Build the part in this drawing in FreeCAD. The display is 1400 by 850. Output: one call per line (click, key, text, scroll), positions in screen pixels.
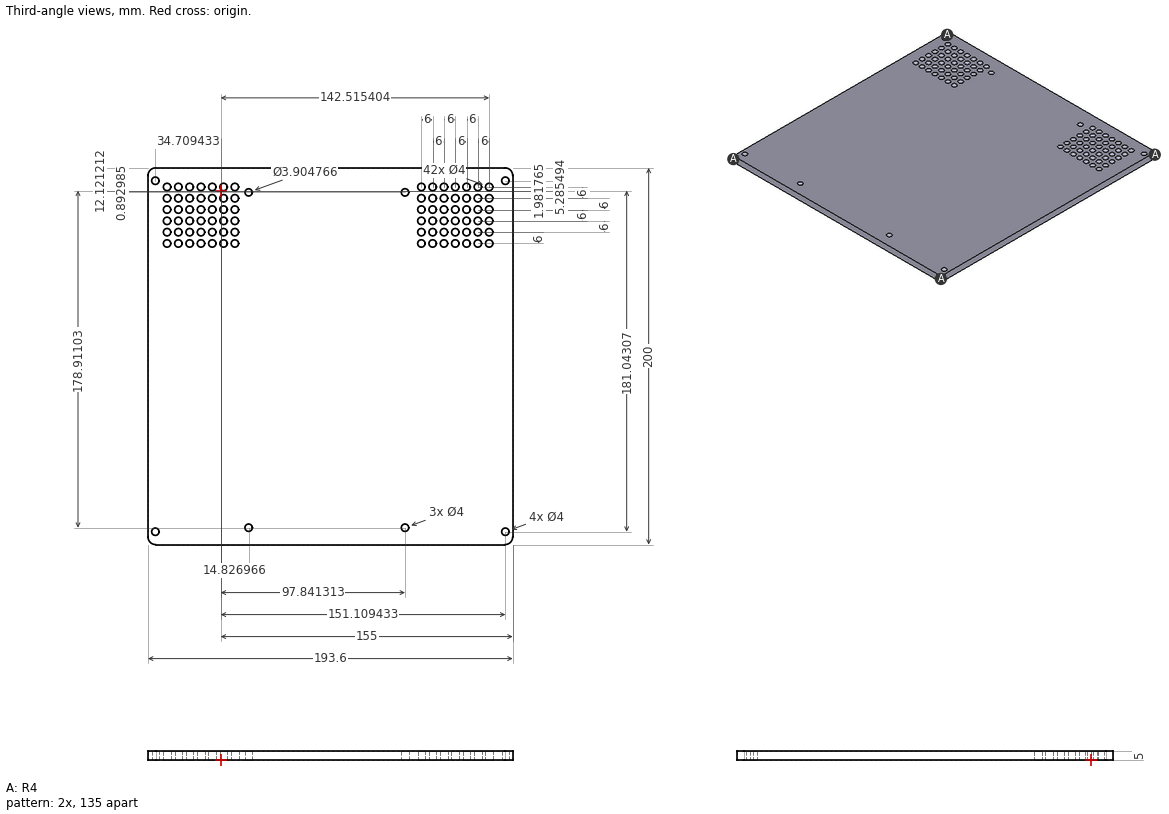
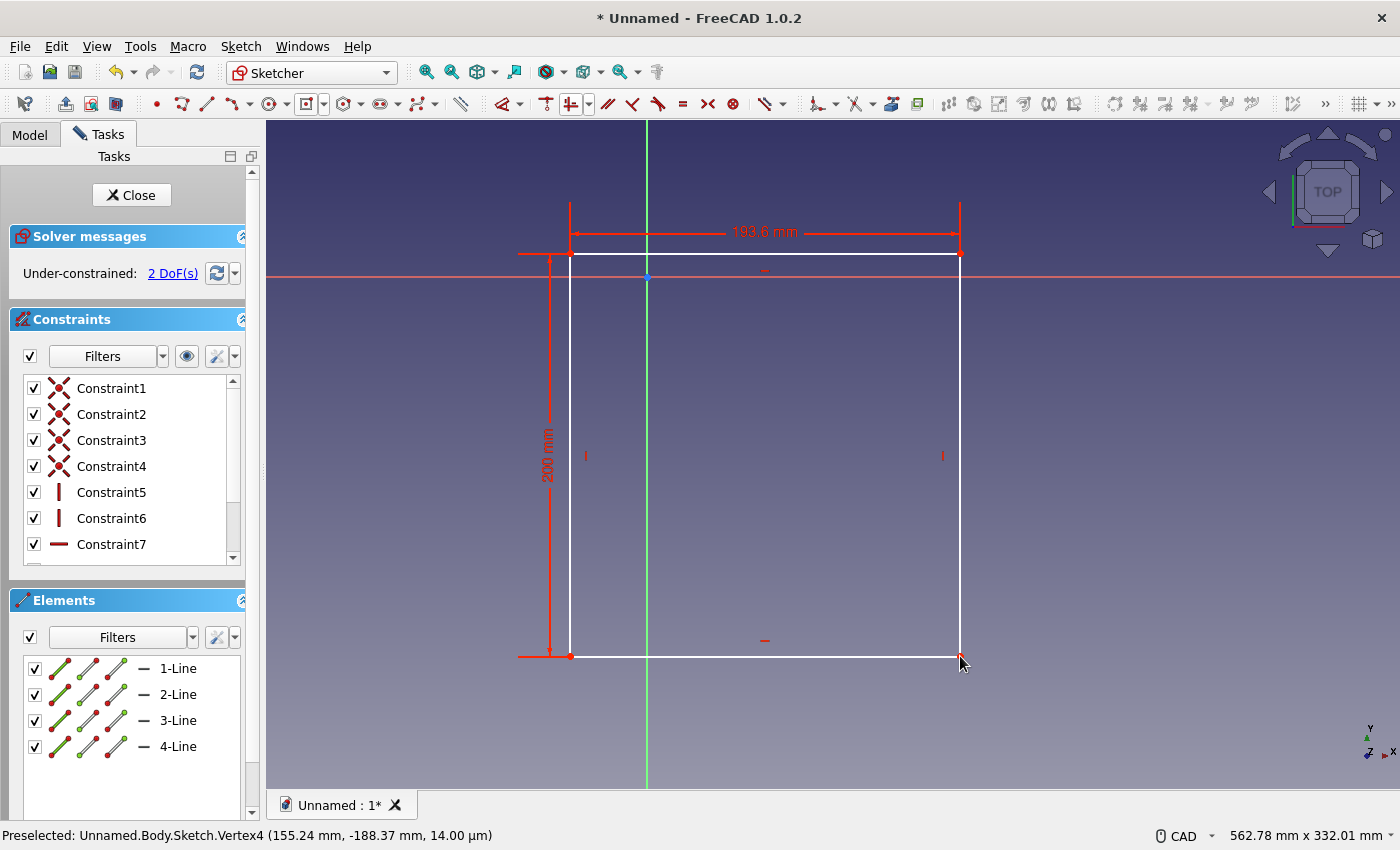
click(502, 104)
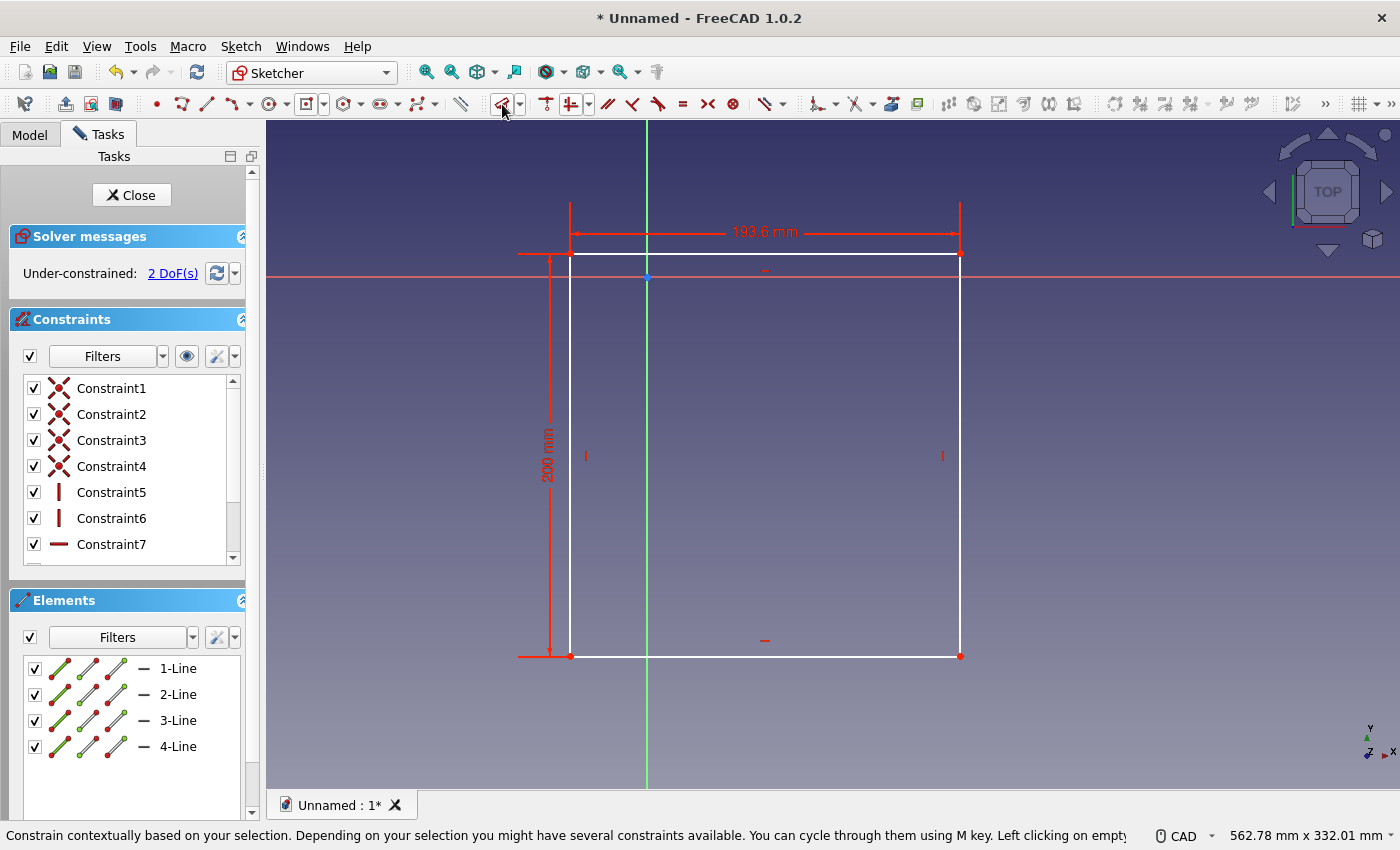
click(960, 657)
click(804, 691)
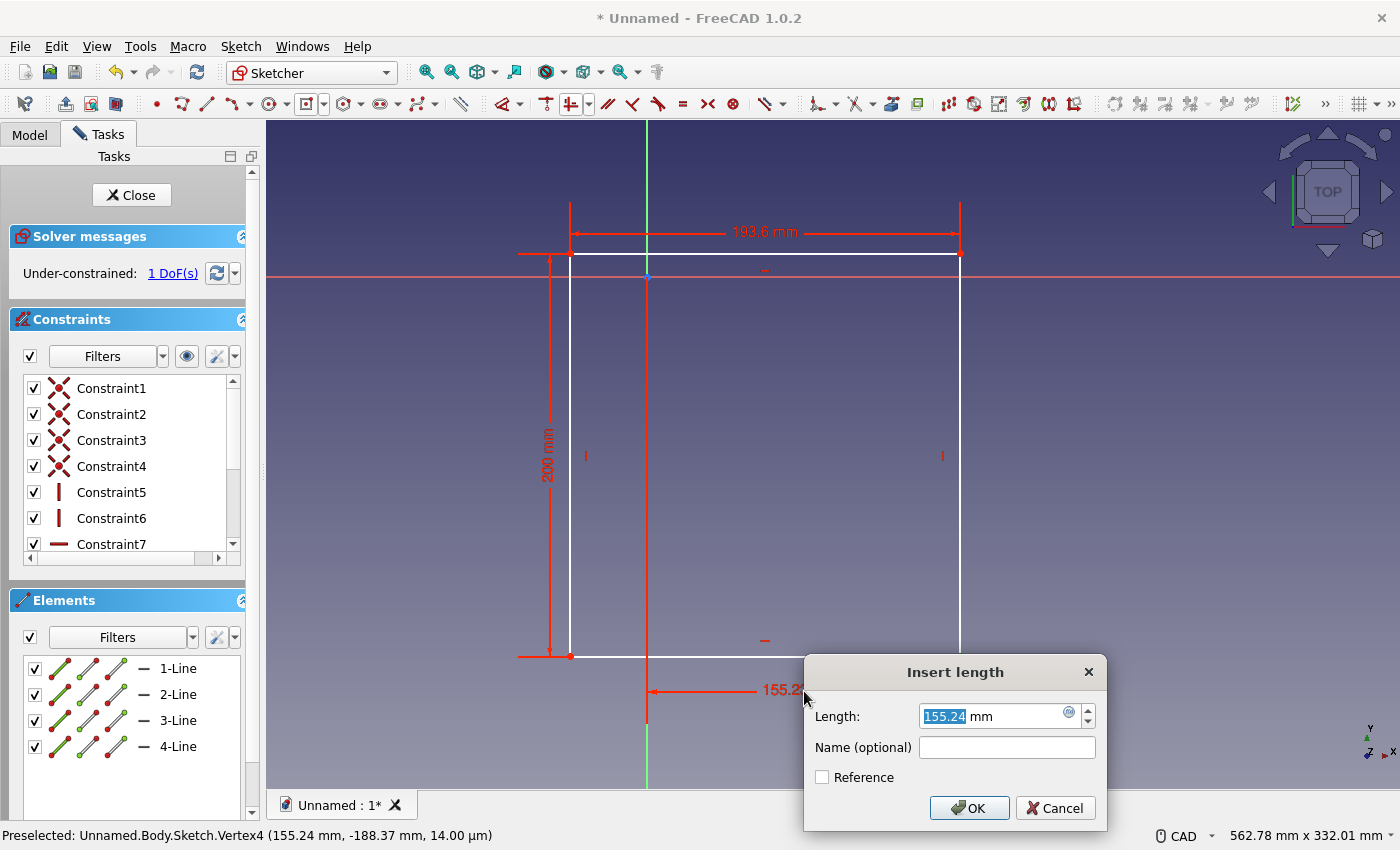
text(155)
key(Return)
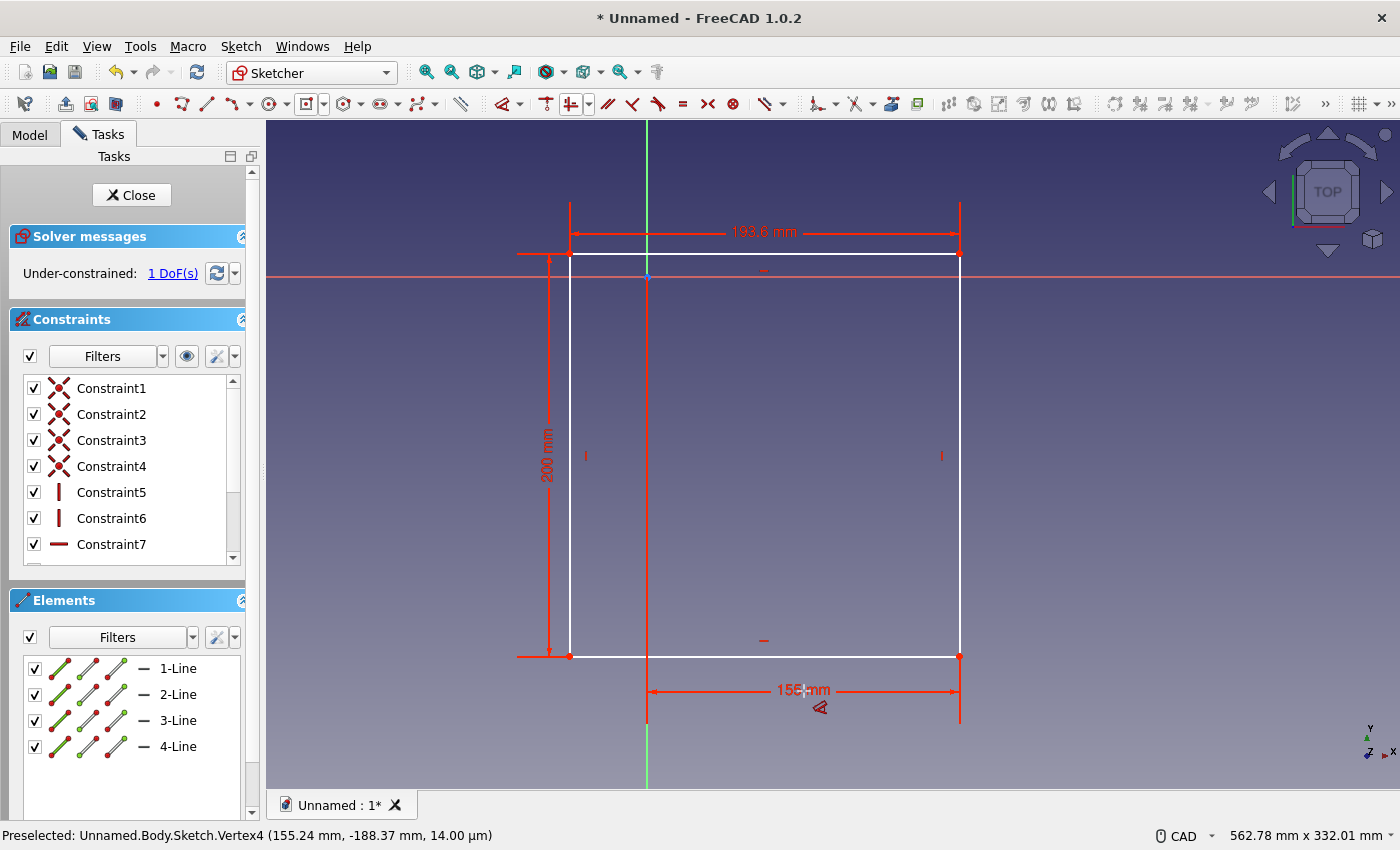
scroll(570, 254, up, 3)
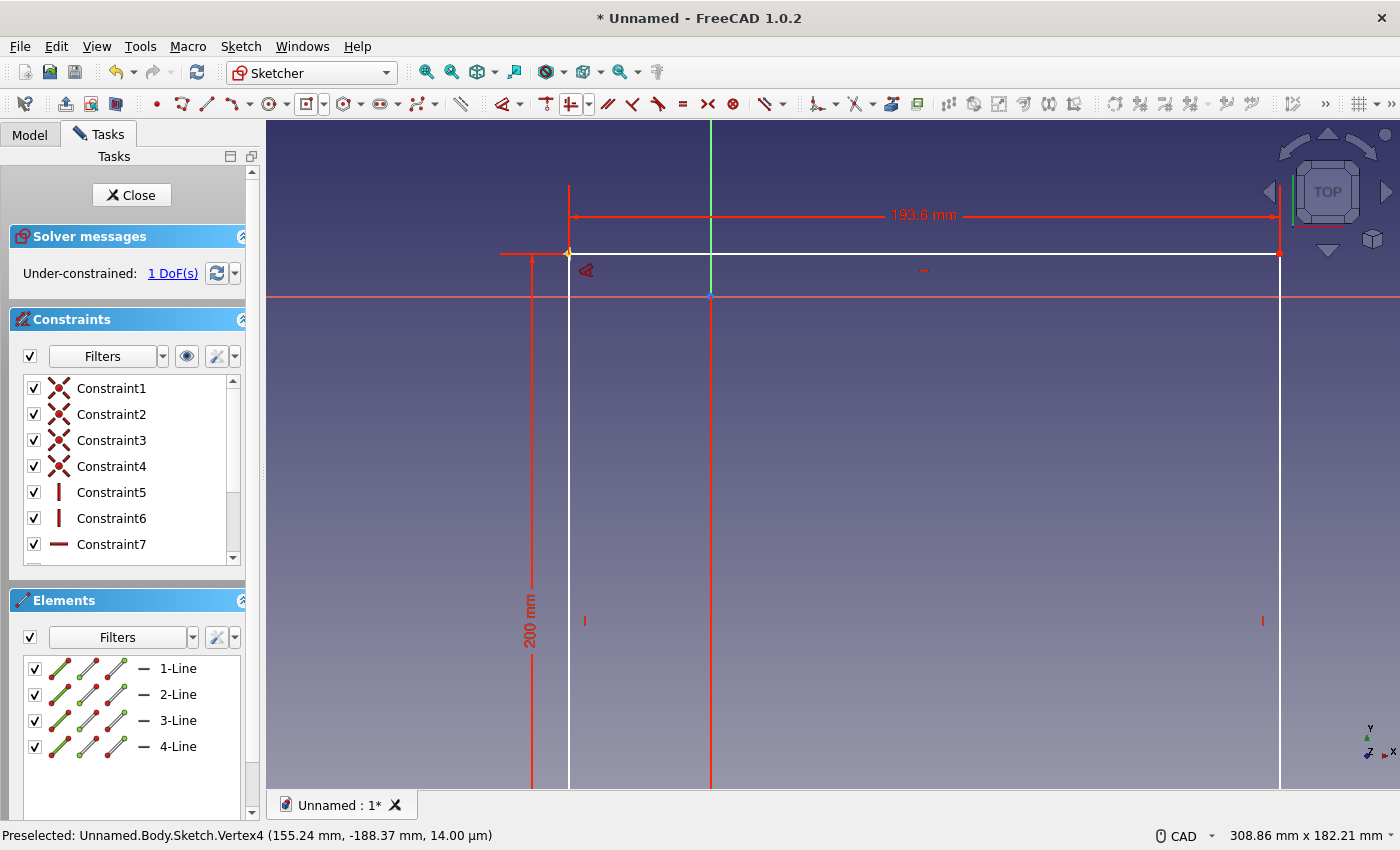
click(569, 254)
click(535, 275)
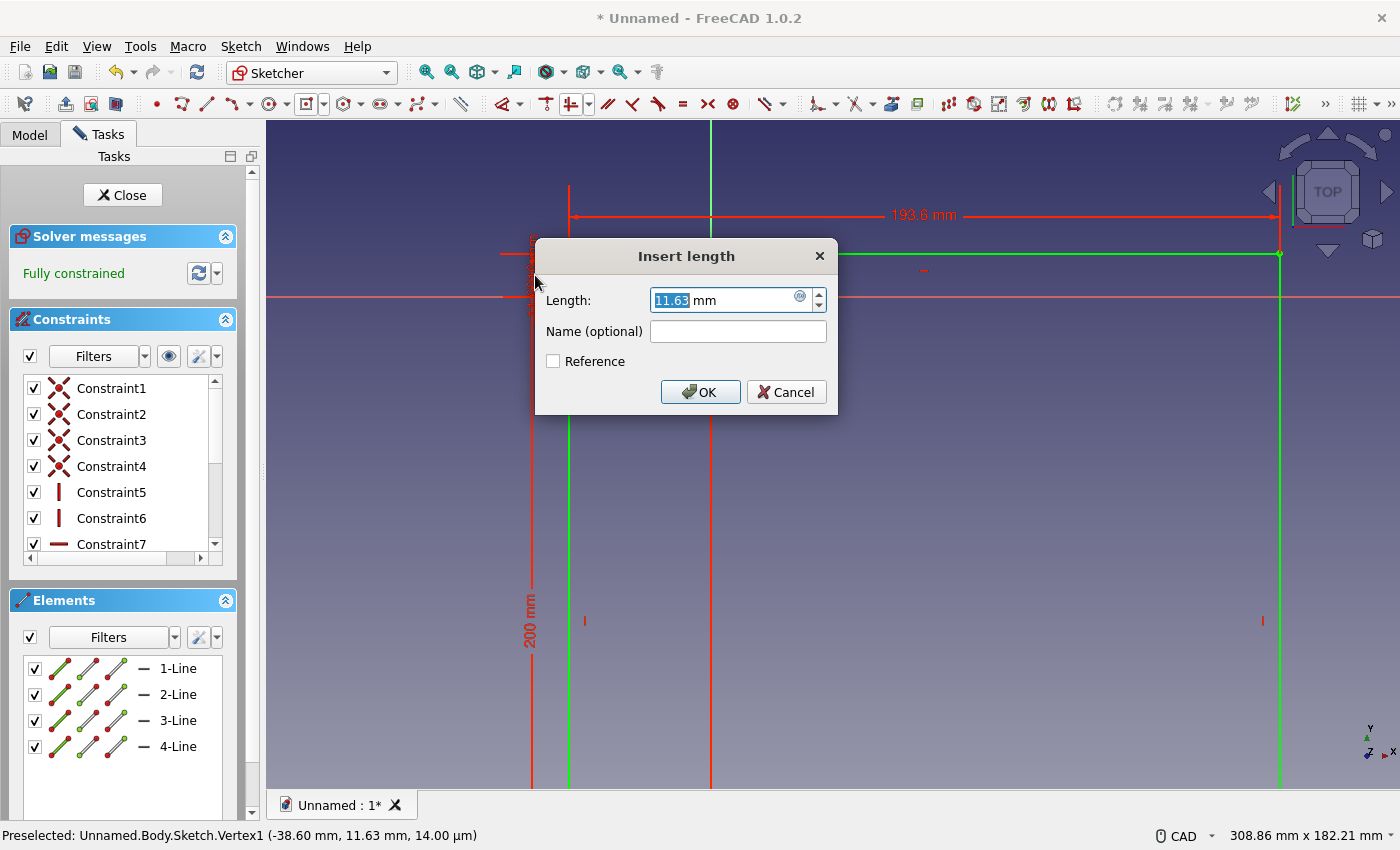
text(12.121212)
key(Return)
key(Escape)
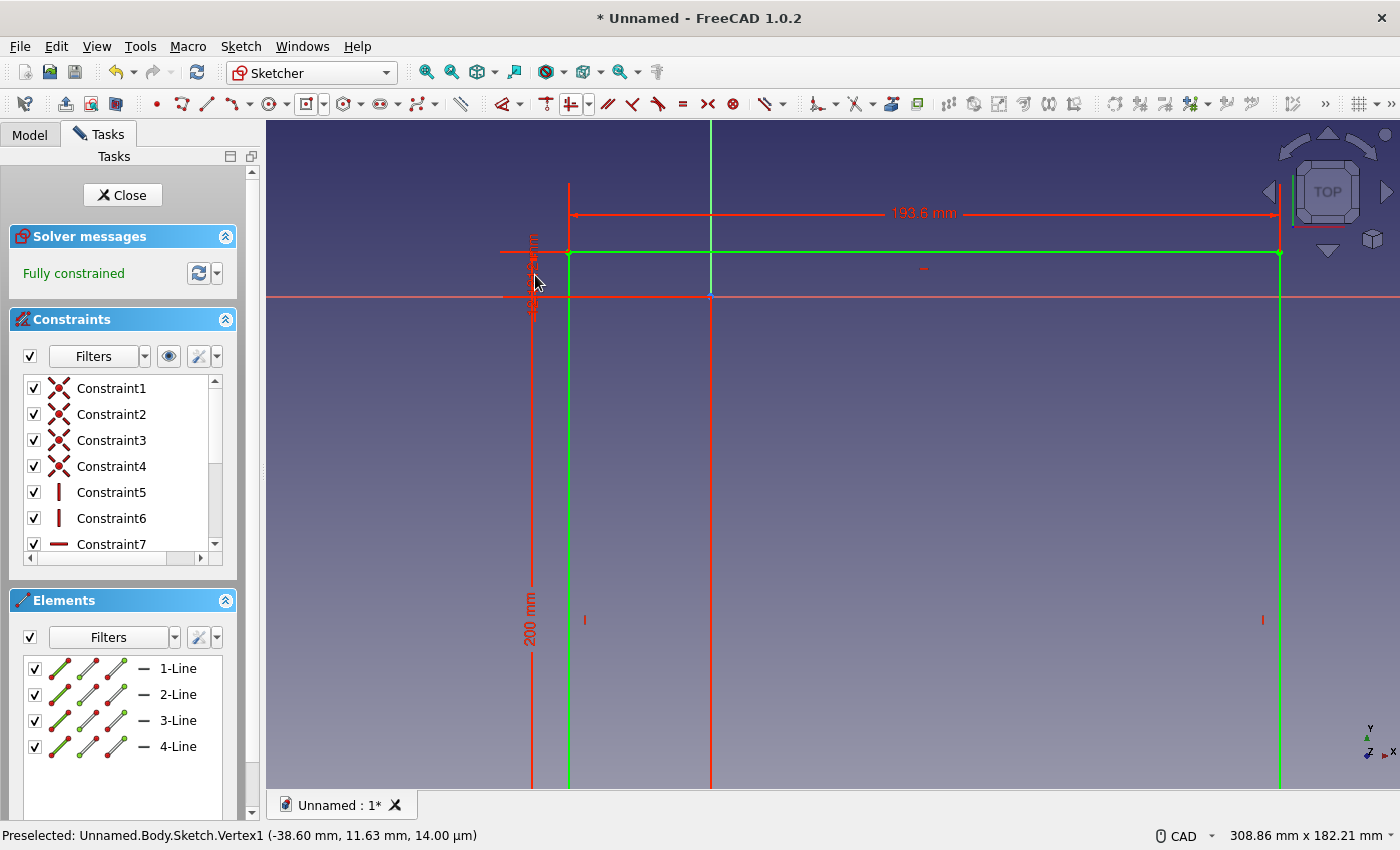
click(123, 195)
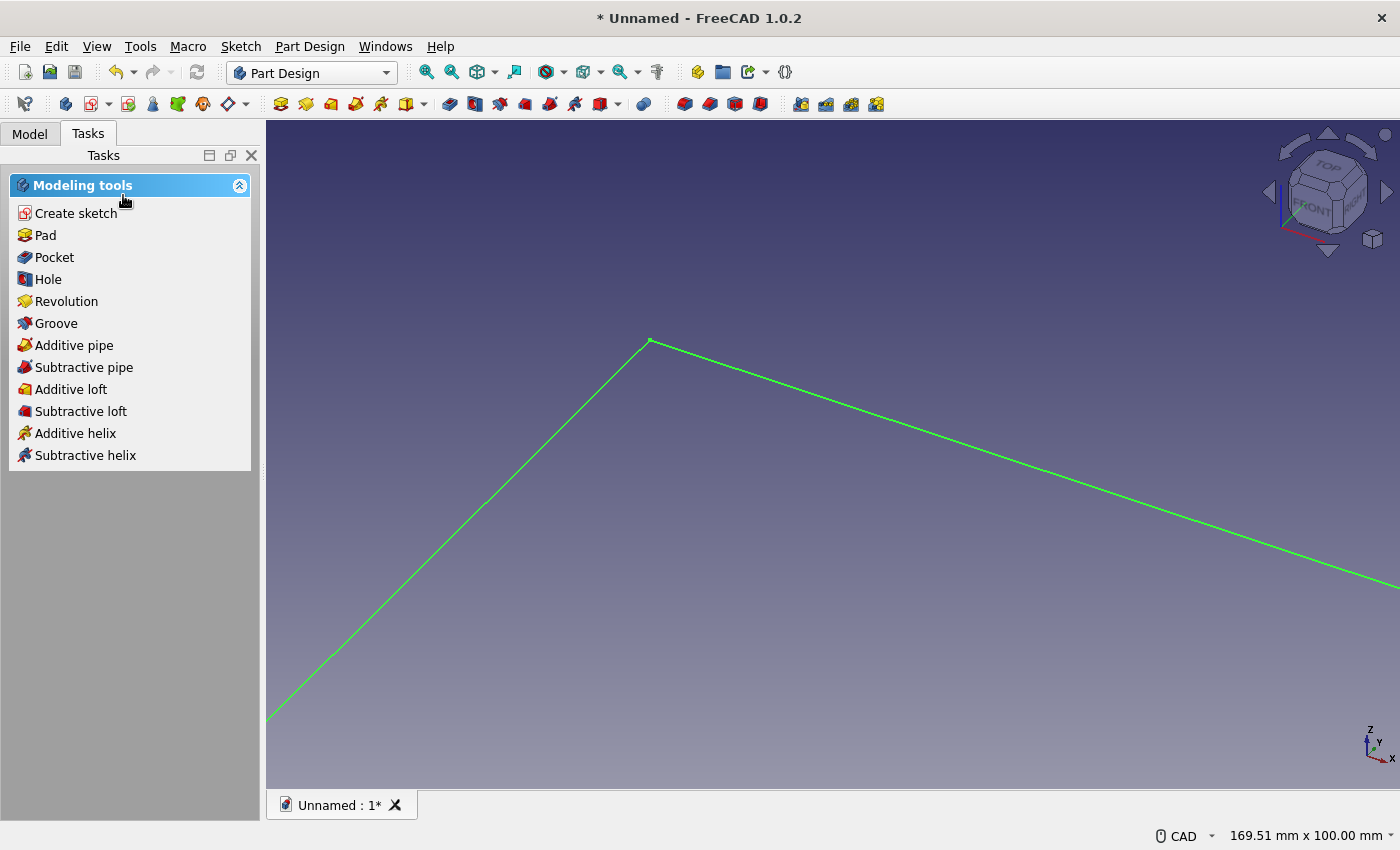
click(281, 104)